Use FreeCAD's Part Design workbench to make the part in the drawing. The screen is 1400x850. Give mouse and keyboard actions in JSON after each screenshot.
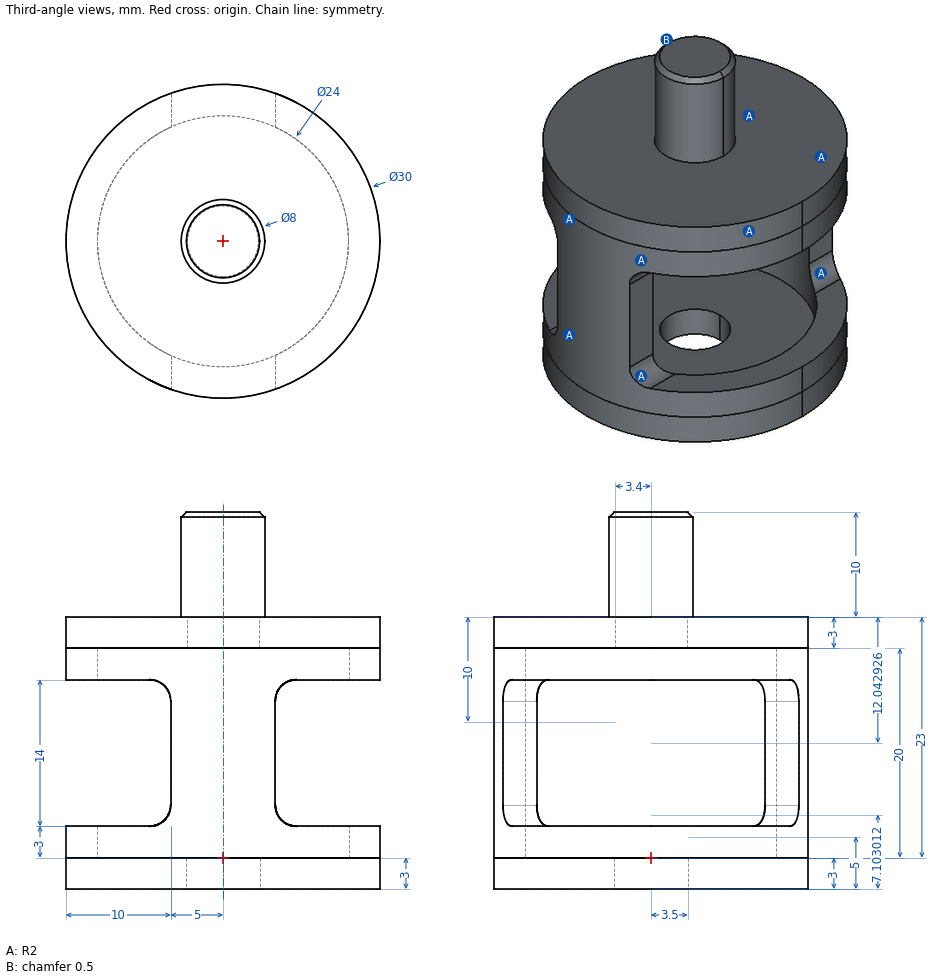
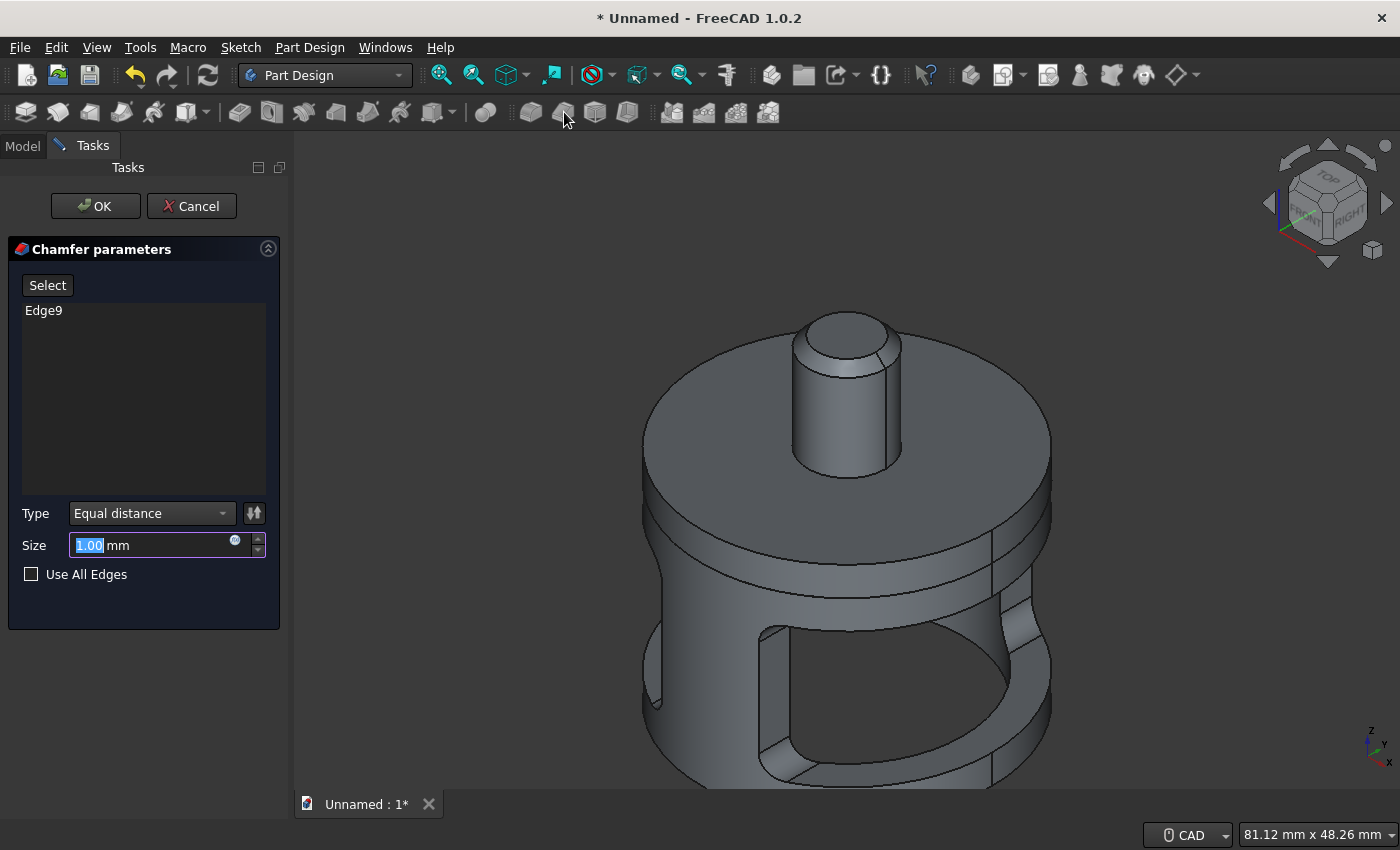
{"action": "type", "text": "0.5"}
{"action": "key", "text": "Tab"}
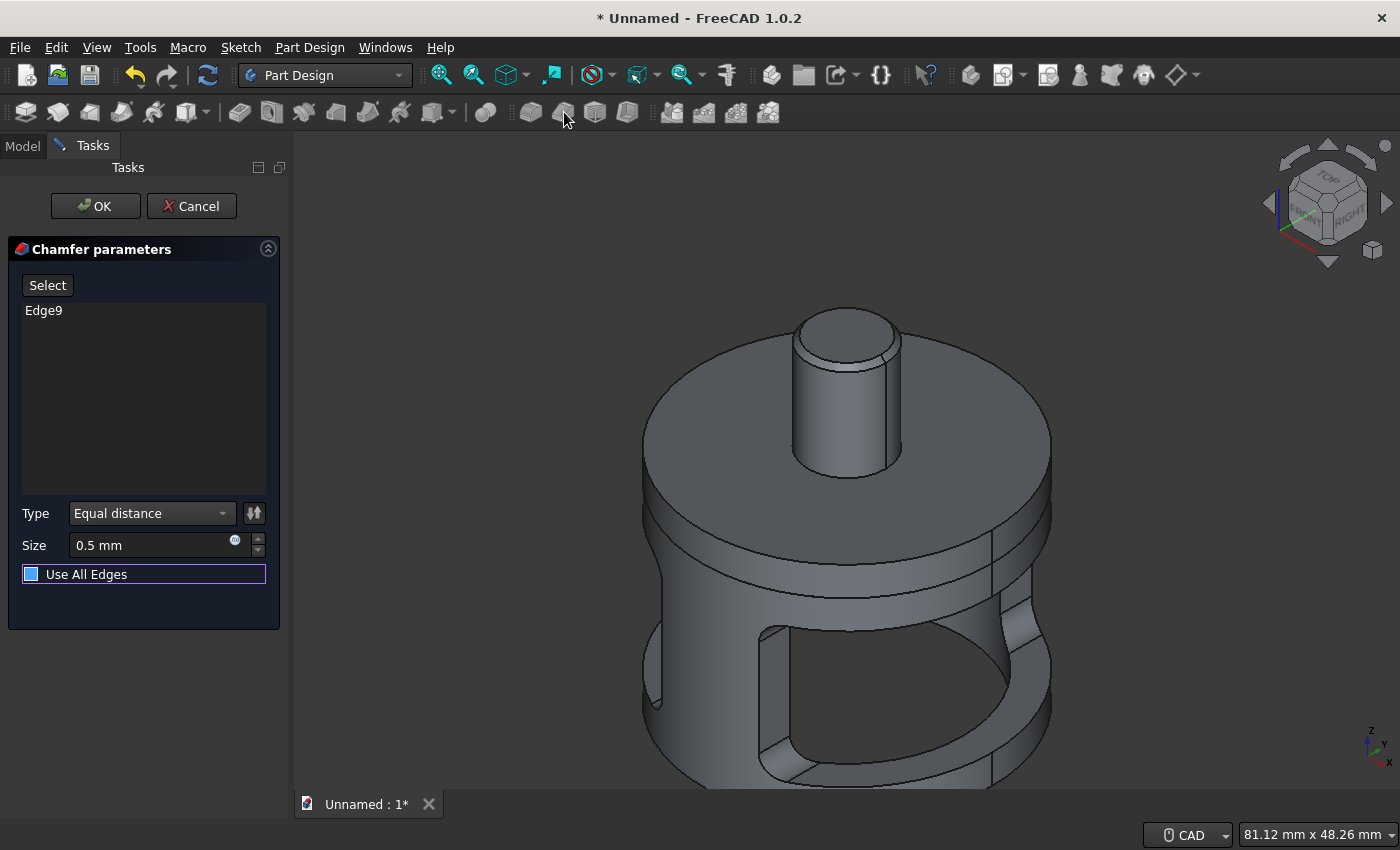
{"action": "left_click", "coordinate": [96, 206]}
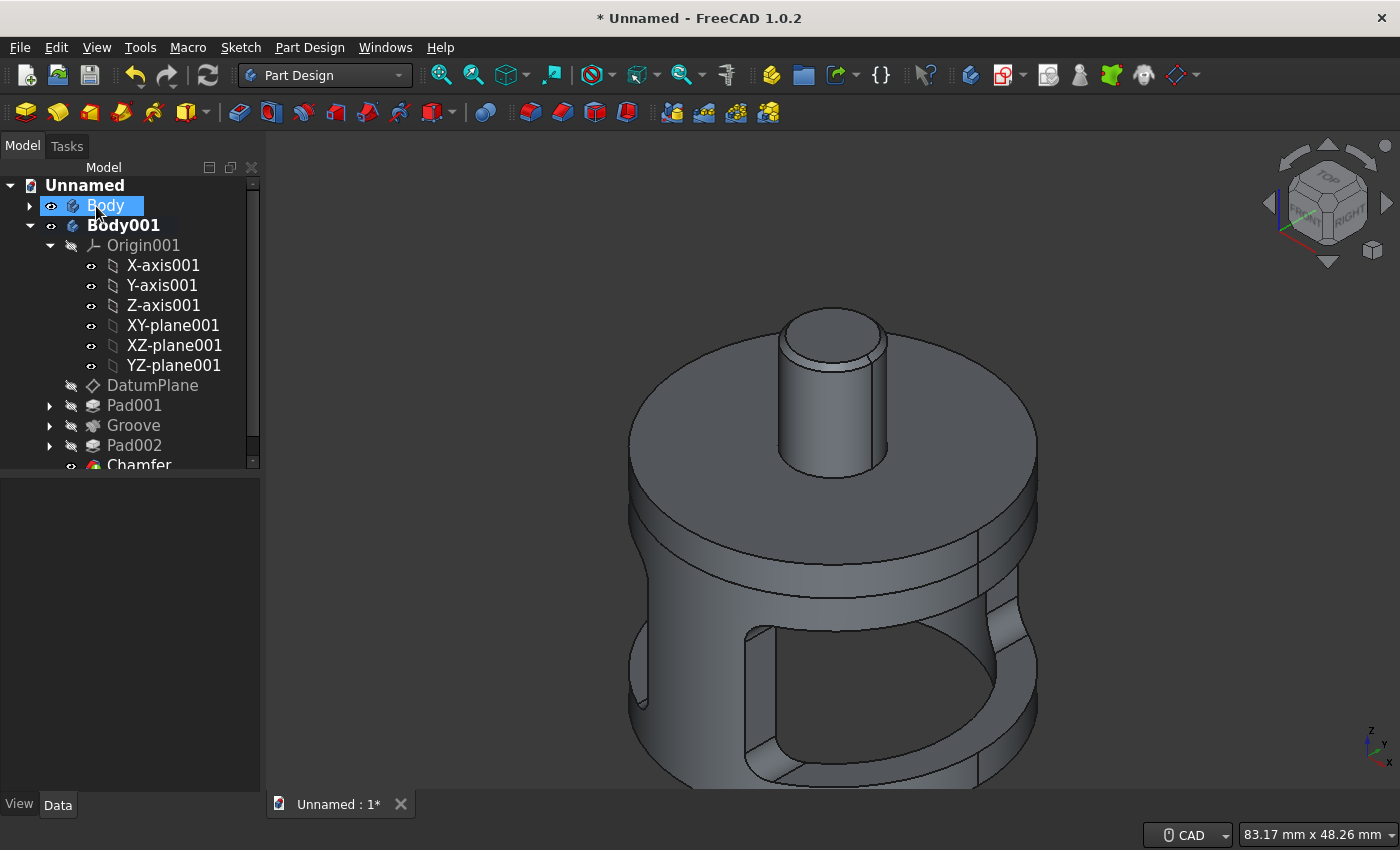
{"action": "left_click", "coordinate": [972, 76]}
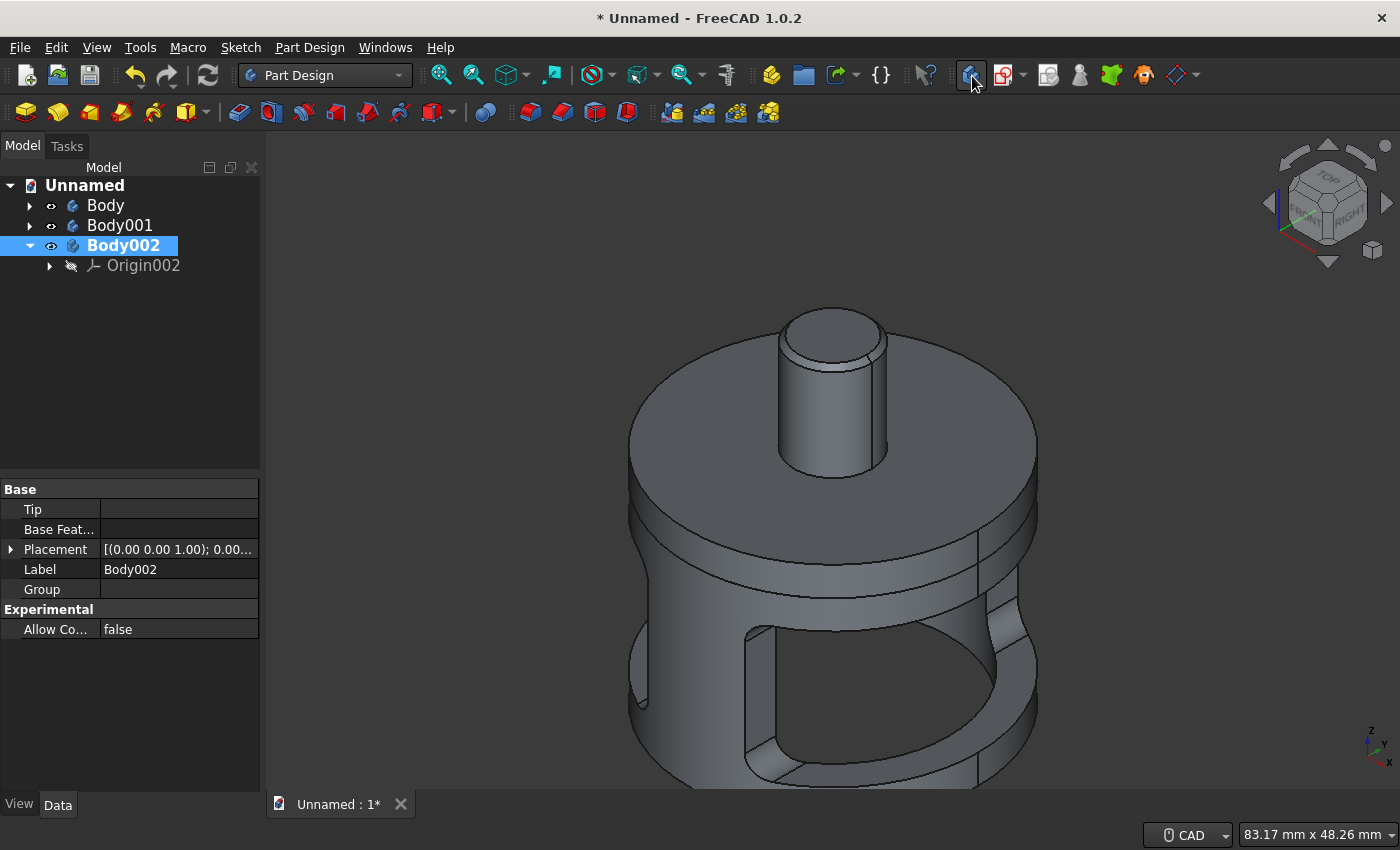
{"action": "left_click", "coordinate": [306, 749]}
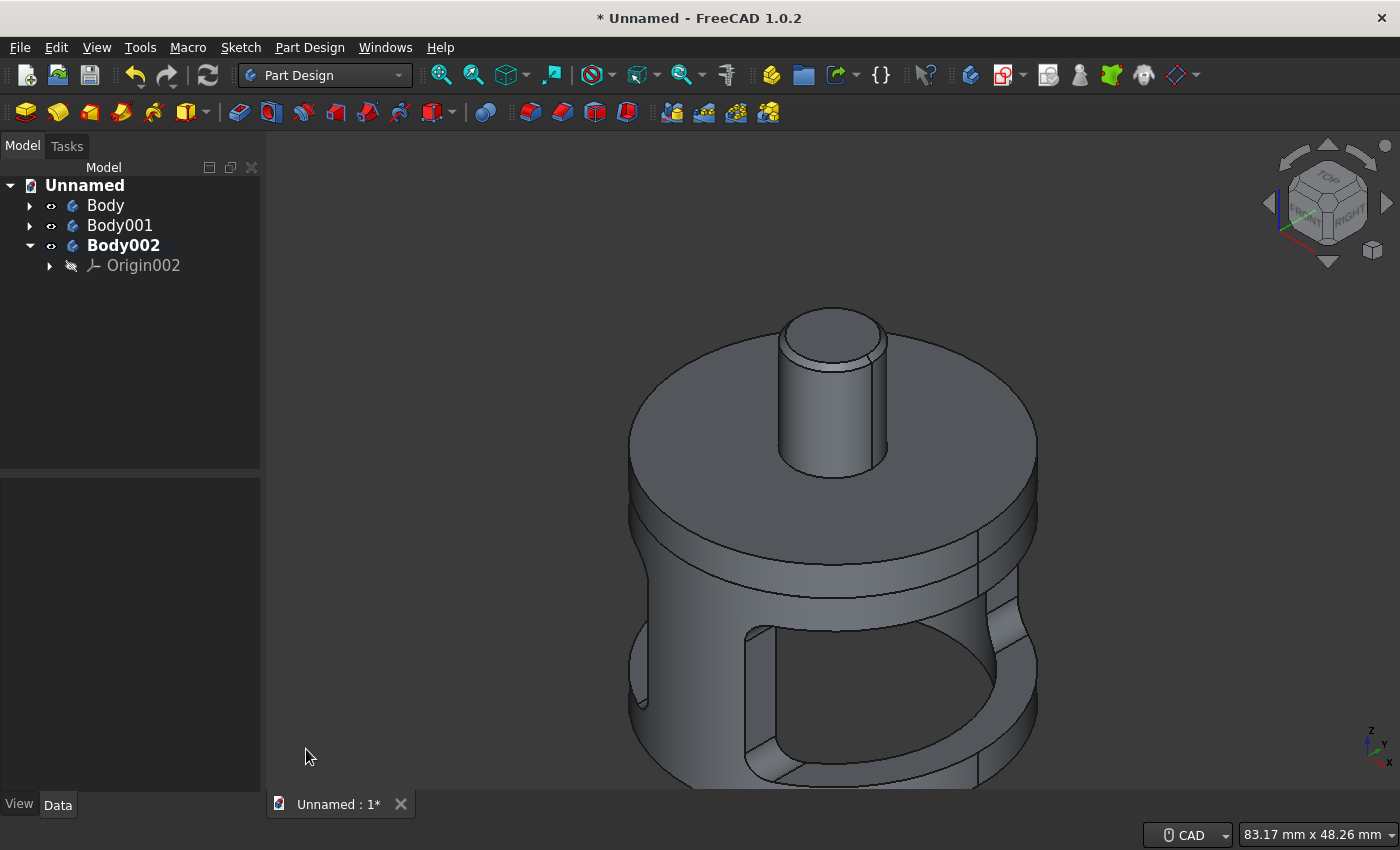
{"action": "left_click", "coordinate": [1004, 76]}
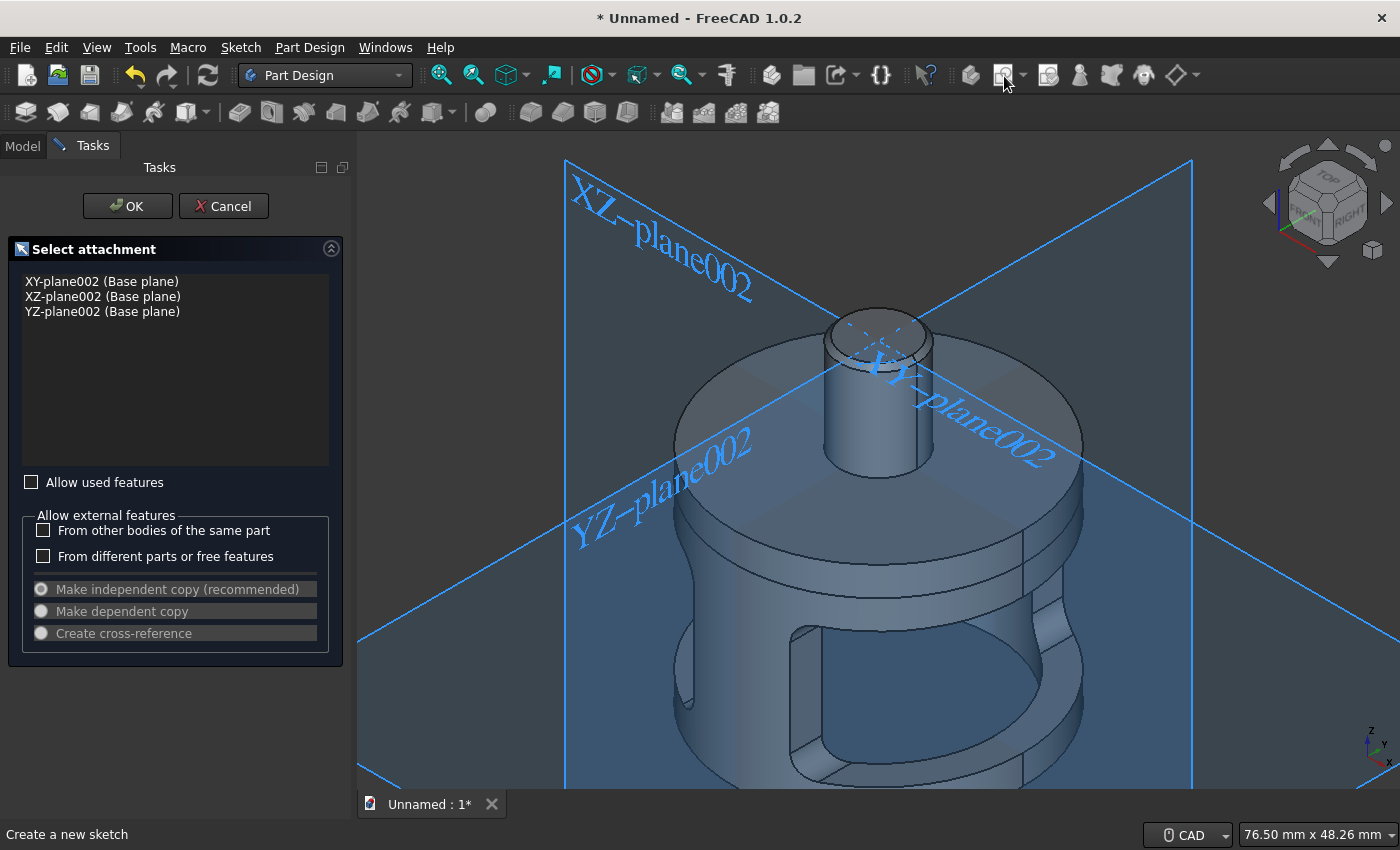
{"action": "left_click", "coordinate": [82, 282]}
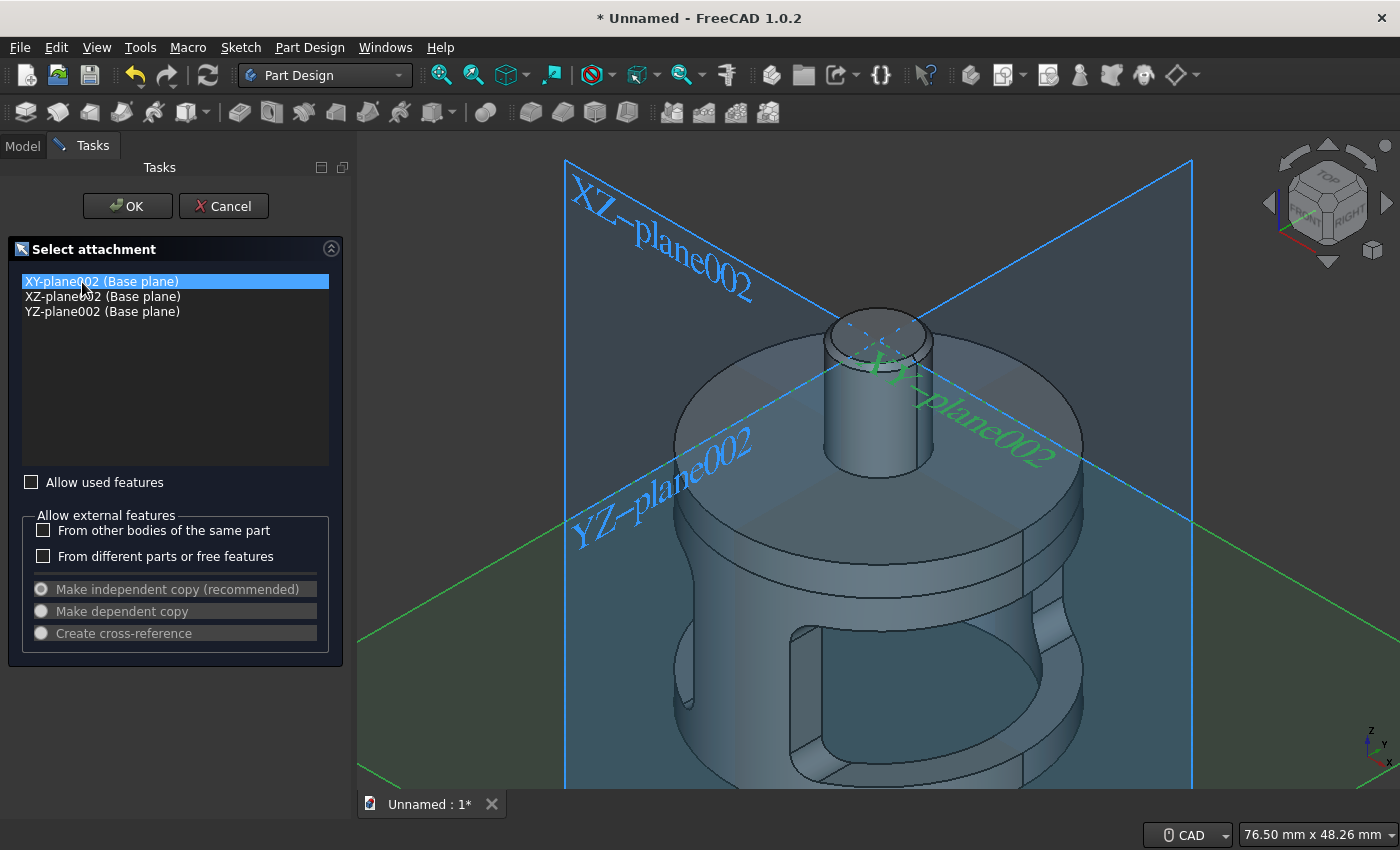
{"action": "left_click", "coordinate": [128, 206]}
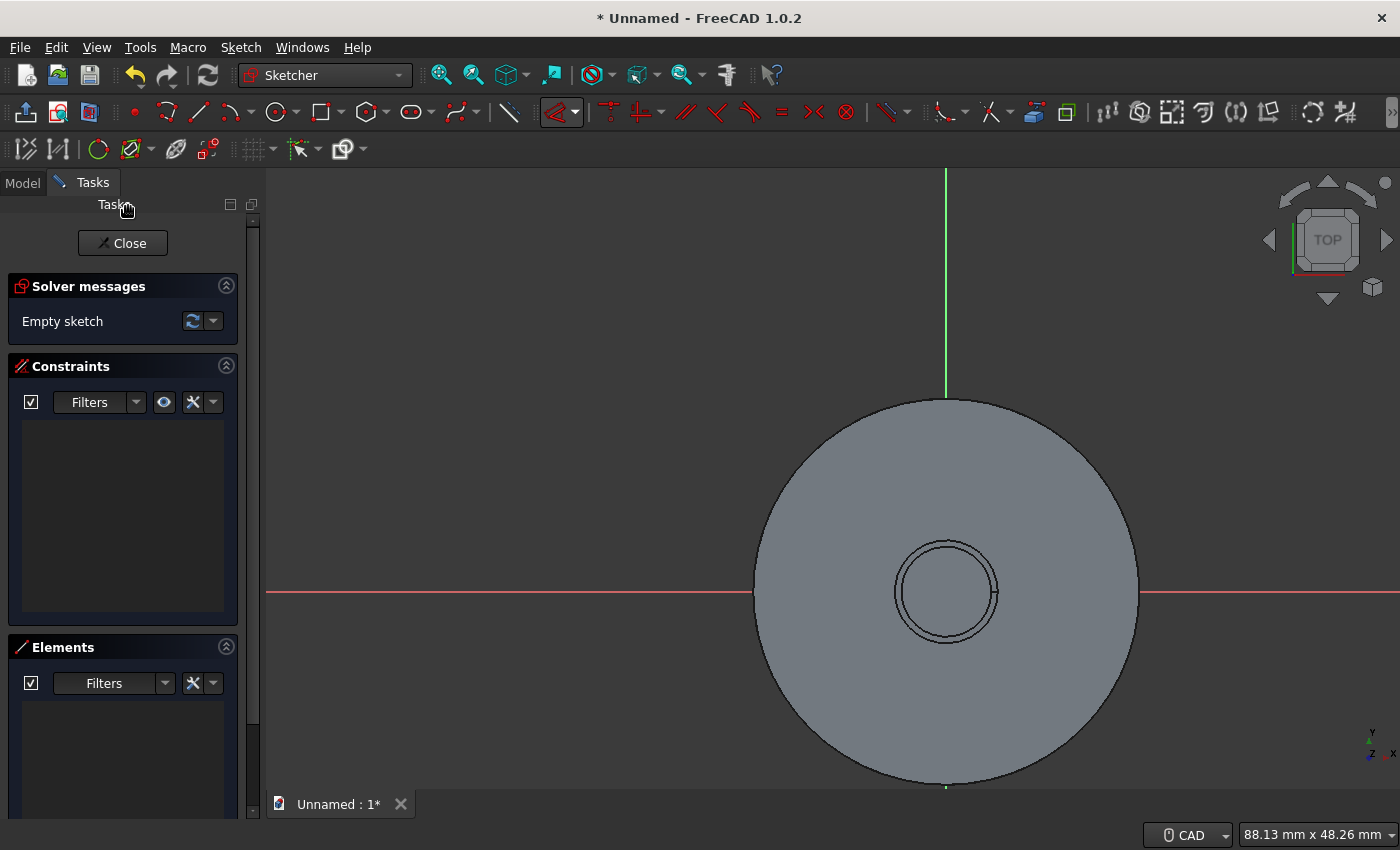
{"action": "scroll", "coordinate": [294, 196], "scroll_direction": "down", "scroll_amount": 1}